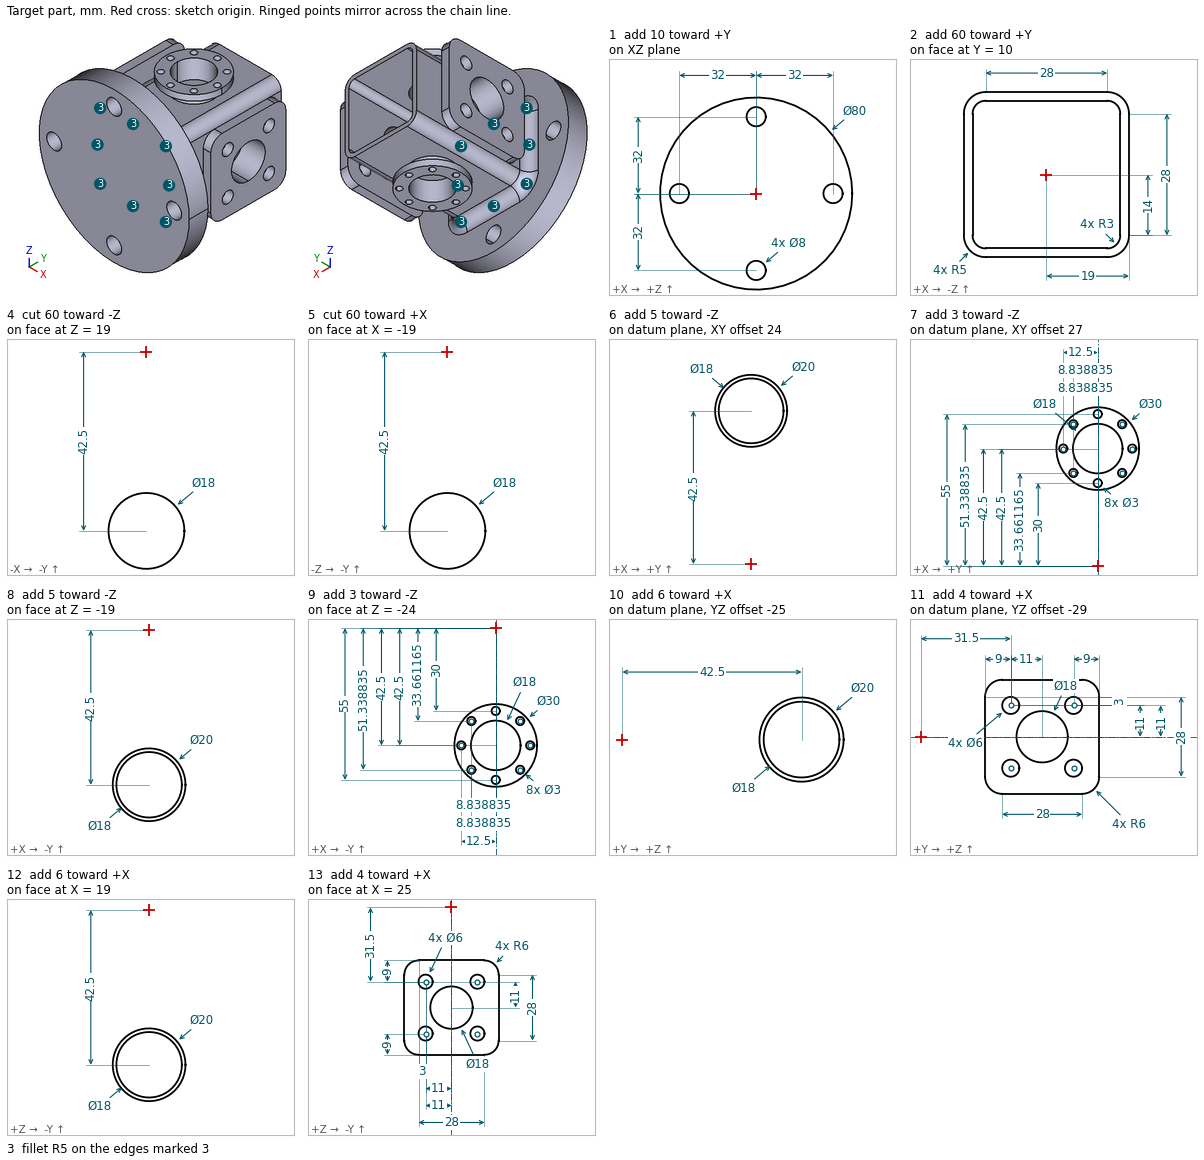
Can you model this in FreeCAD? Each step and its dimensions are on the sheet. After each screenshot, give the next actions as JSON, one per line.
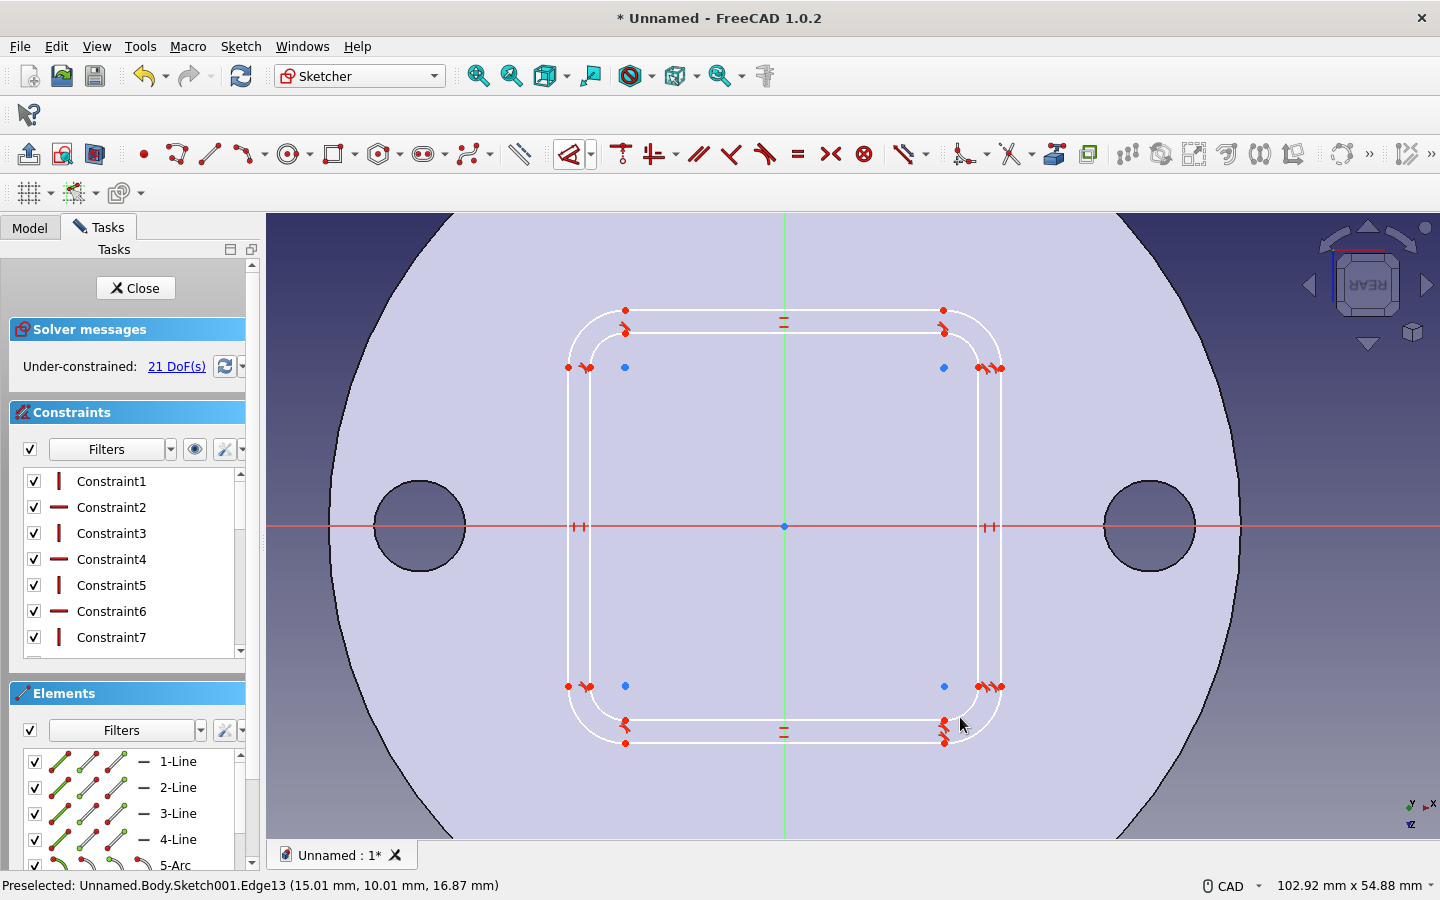
{"action": "left_click", "coordinate": [849, 720]}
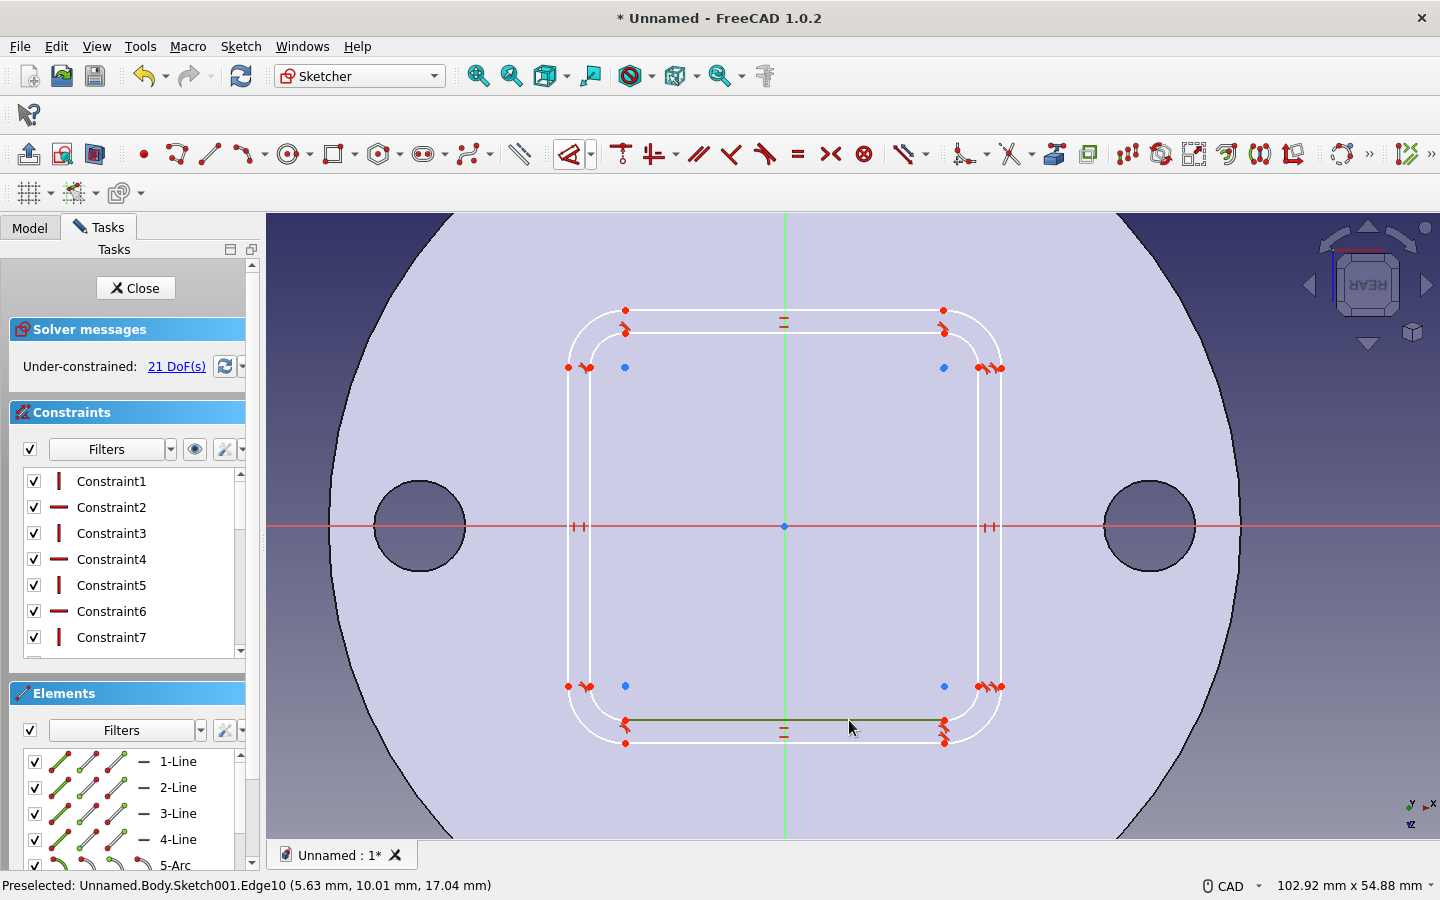
{"action": "left_click", "coordinate": [595, 702]}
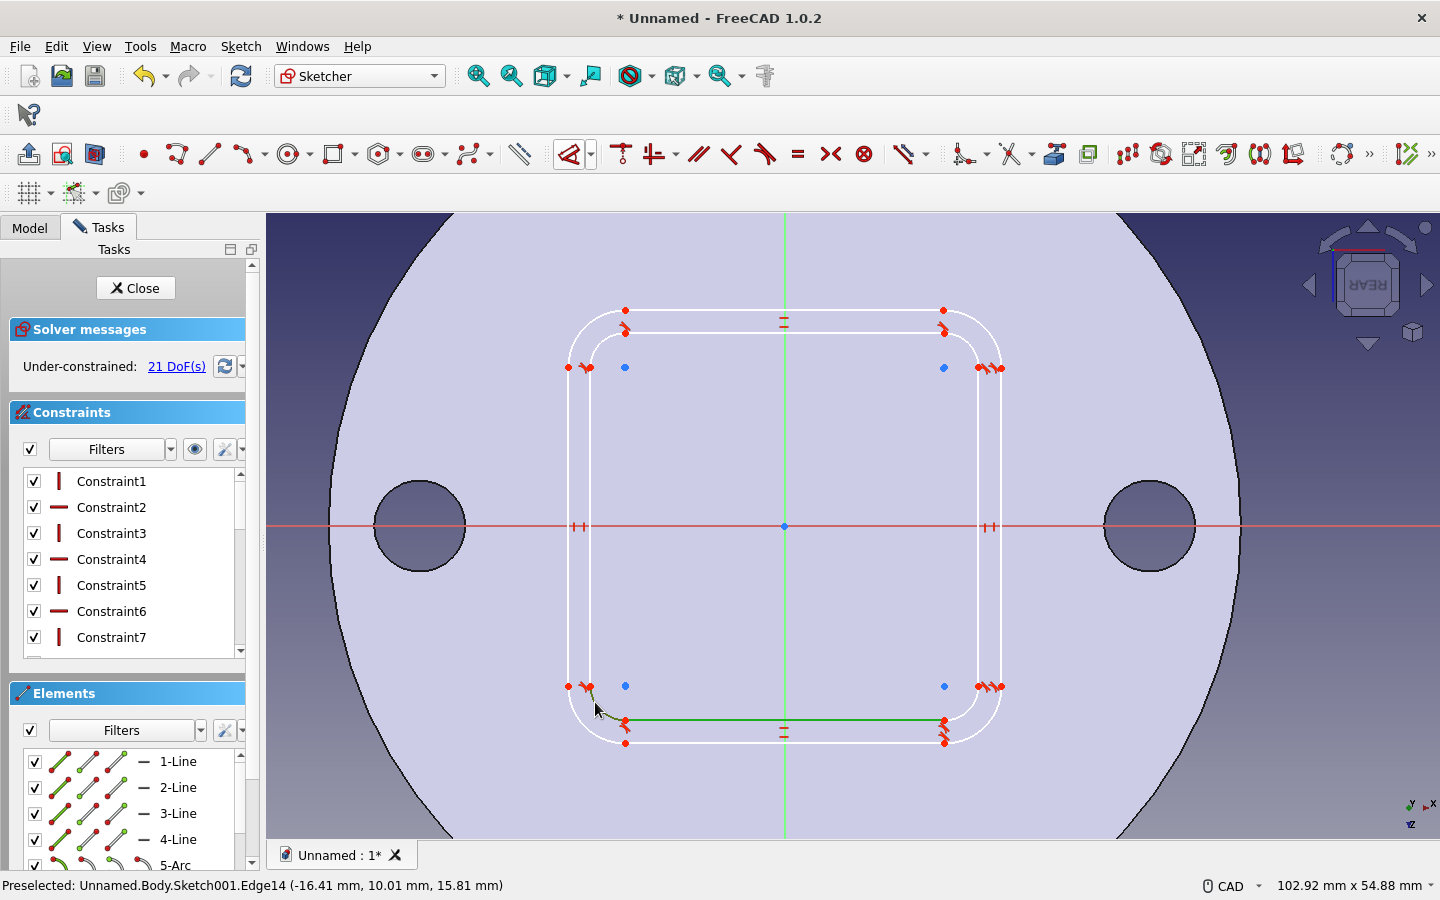
{"action": "left_click", "coordinate": [765, 154]}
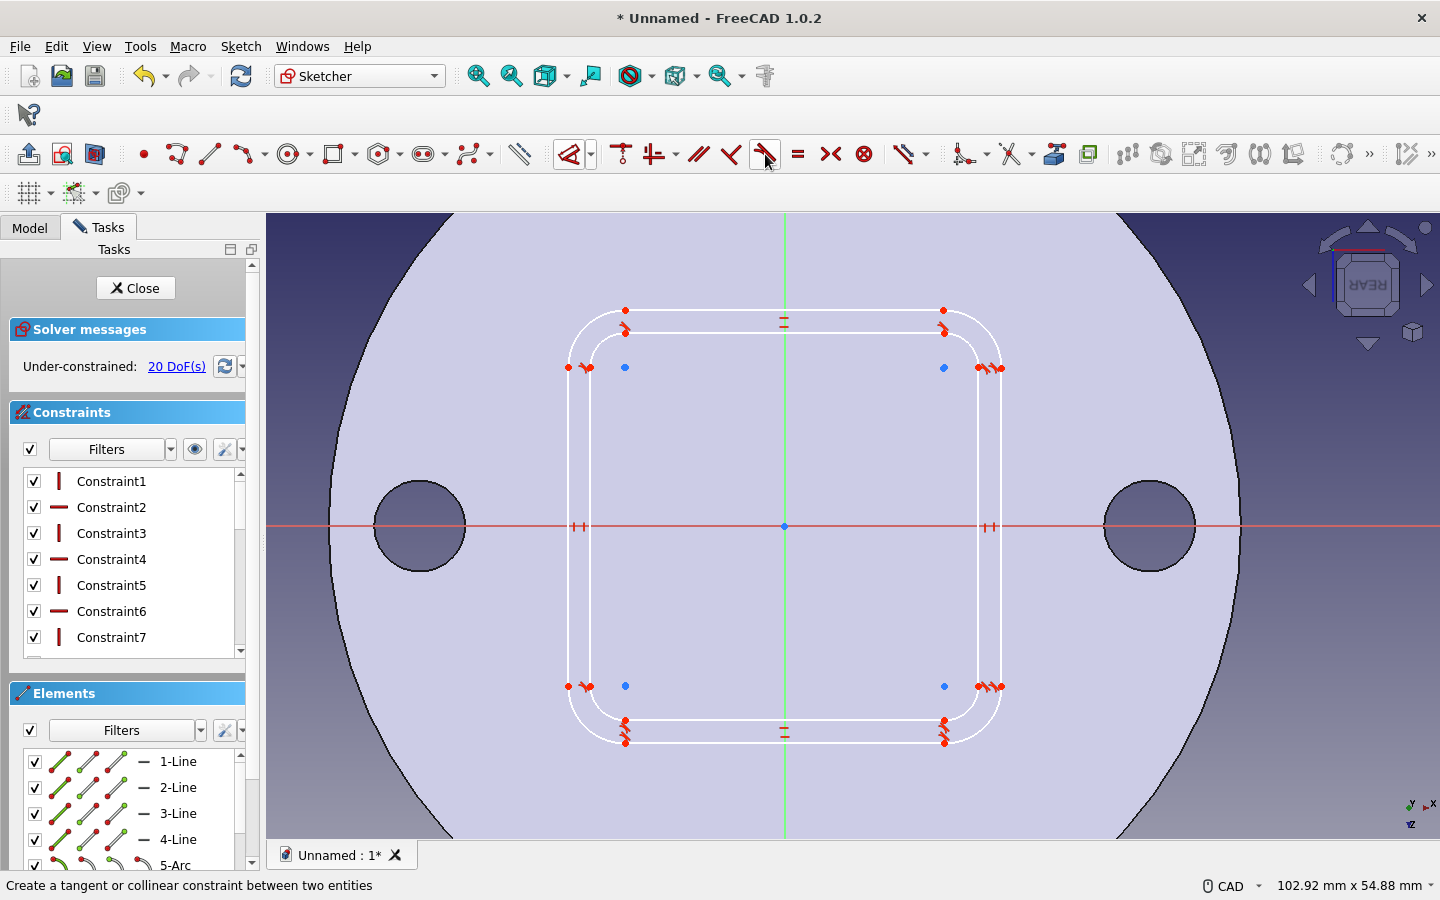
{"action": "left_click", "coordinate": [590, 591]}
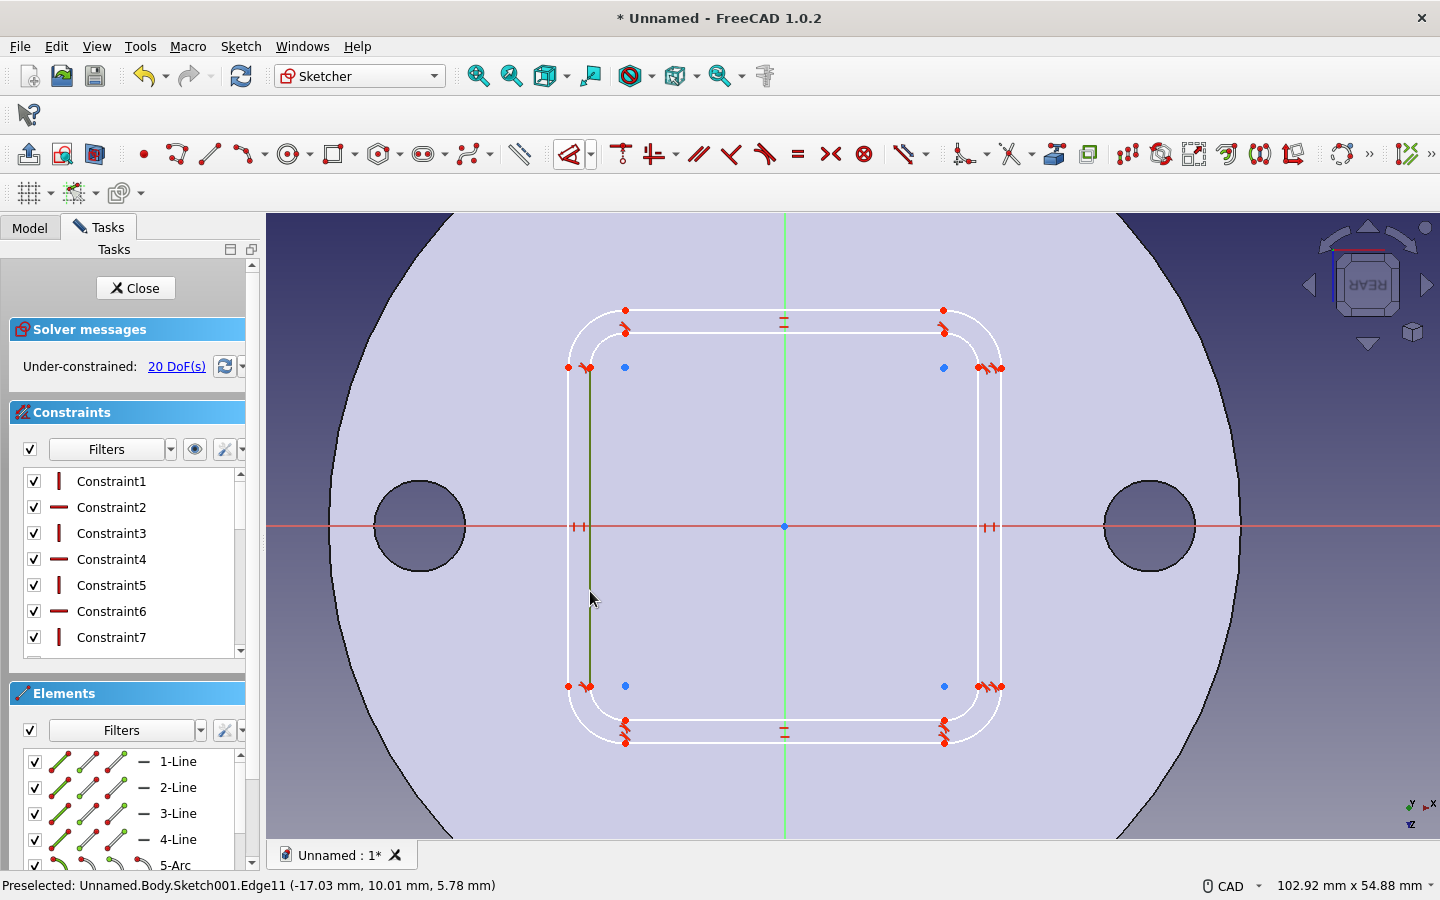
{"action": "left_click", "coordinate": [595, 702]}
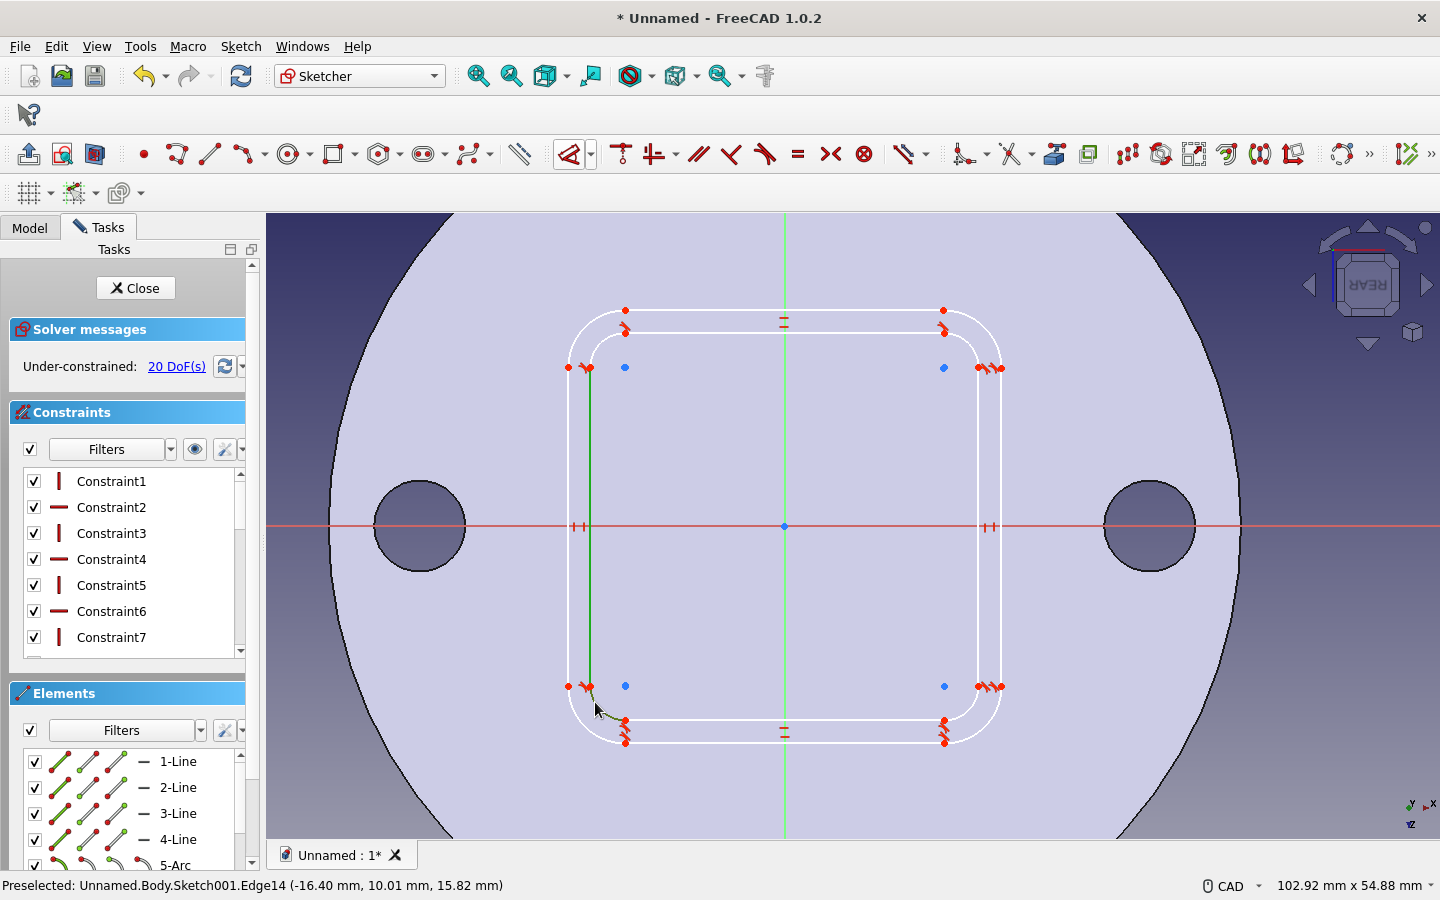
{"action": "key", "text": "t"}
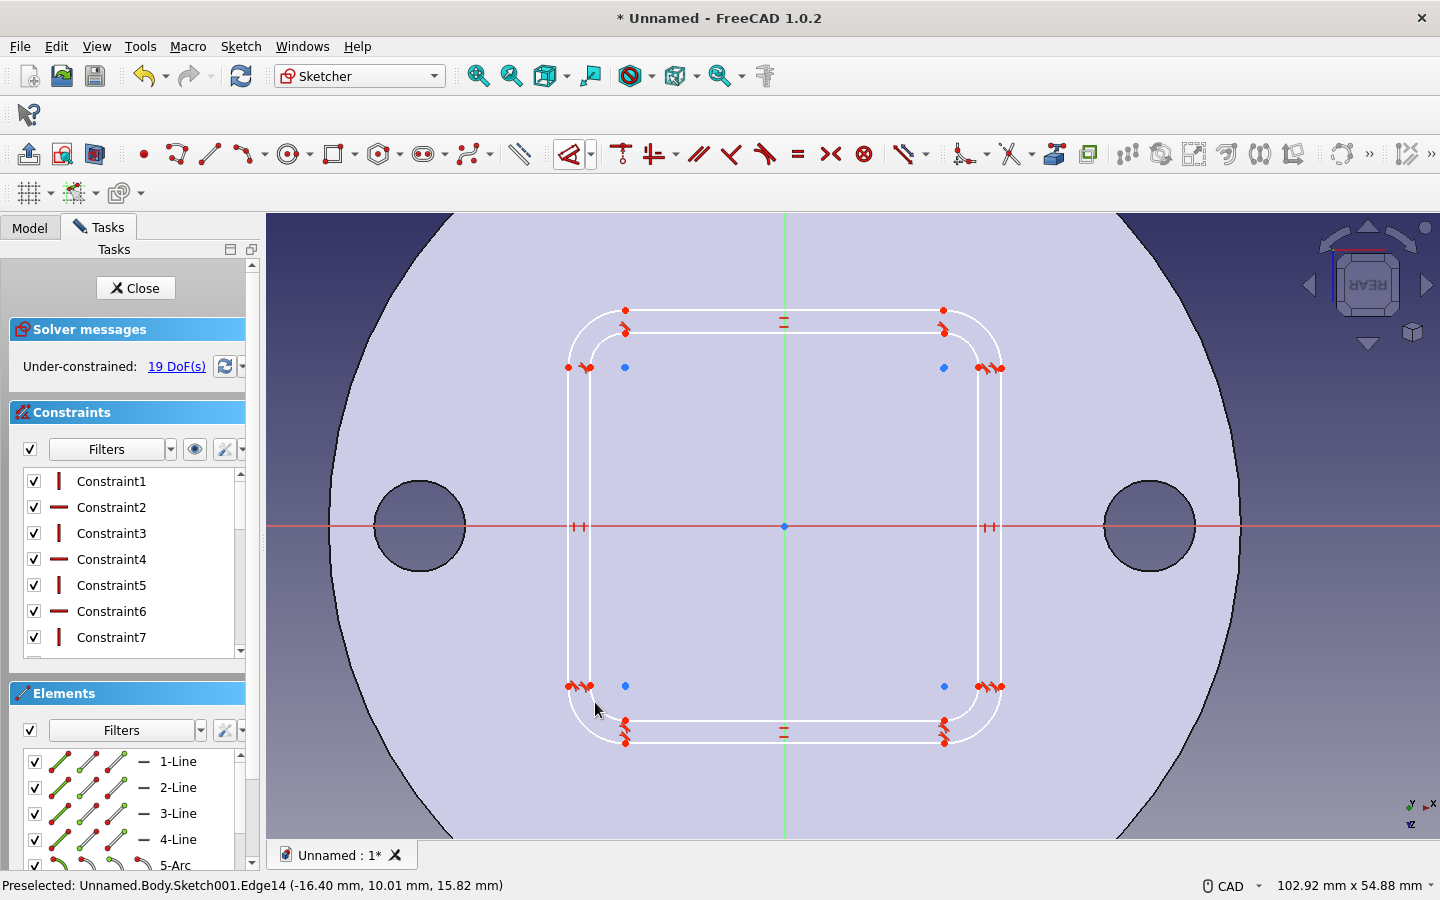
{"action": "left_click", "coordinate": [590, 590]}